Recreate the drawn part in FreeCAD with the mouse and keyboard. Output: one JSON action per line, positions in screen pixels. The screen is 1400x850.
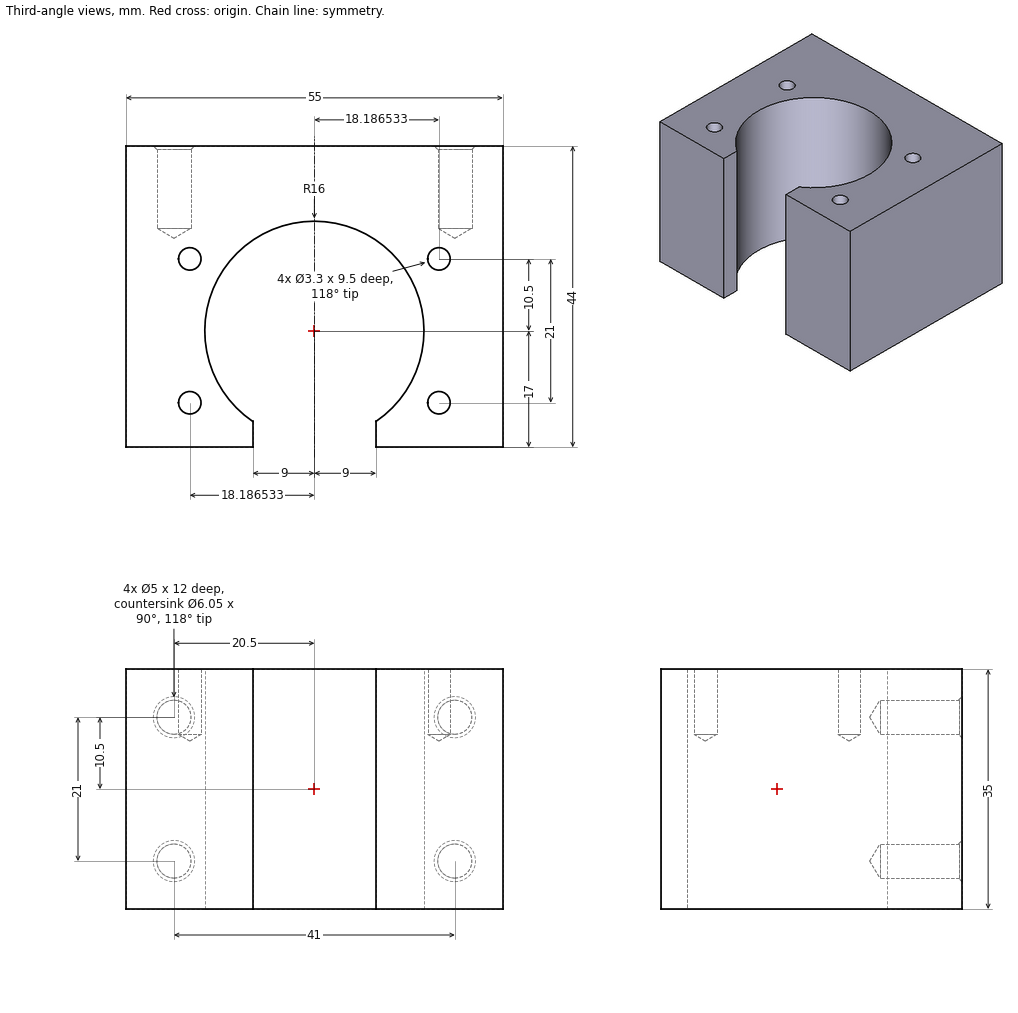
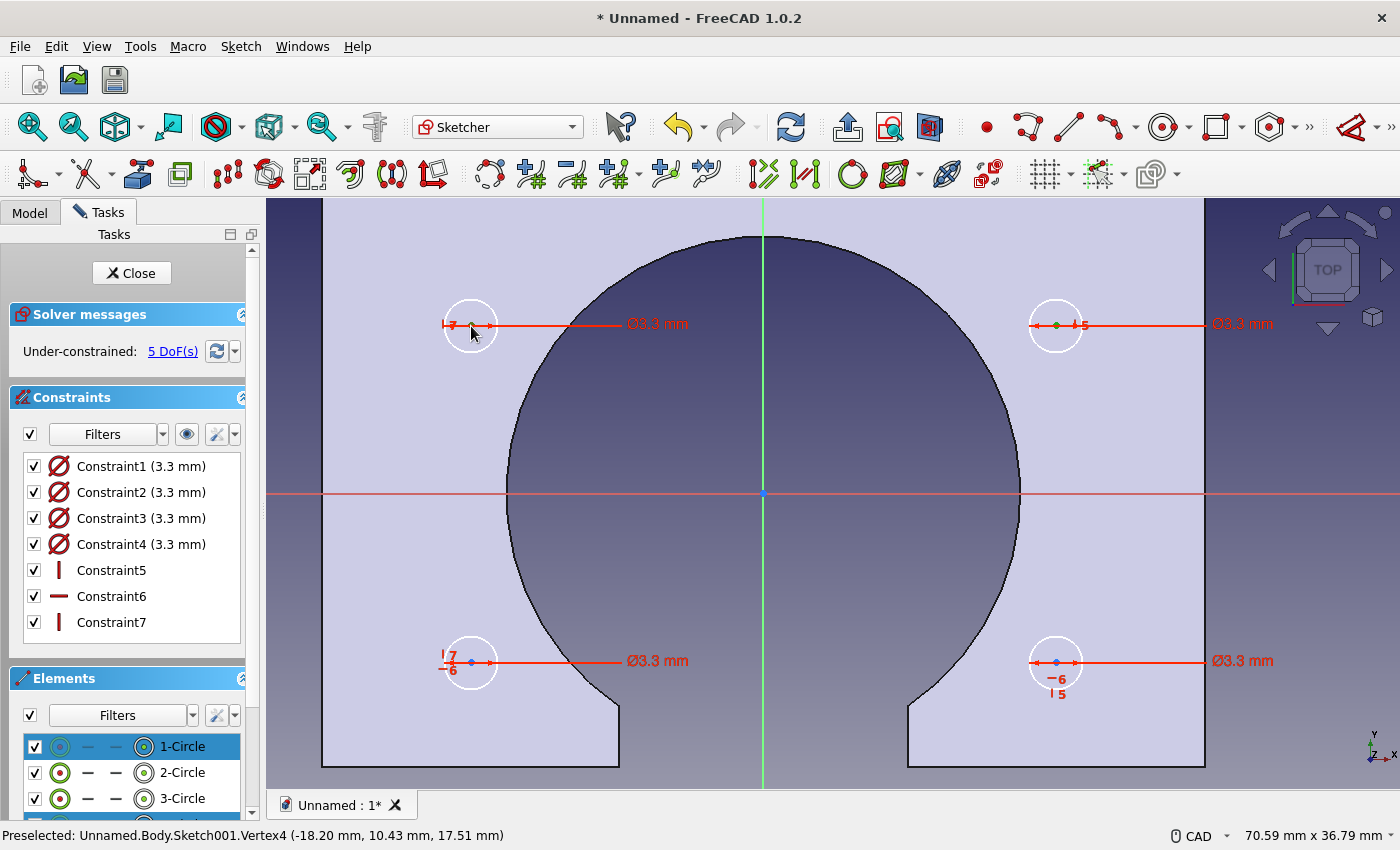
{"action": "key", "text": "h"}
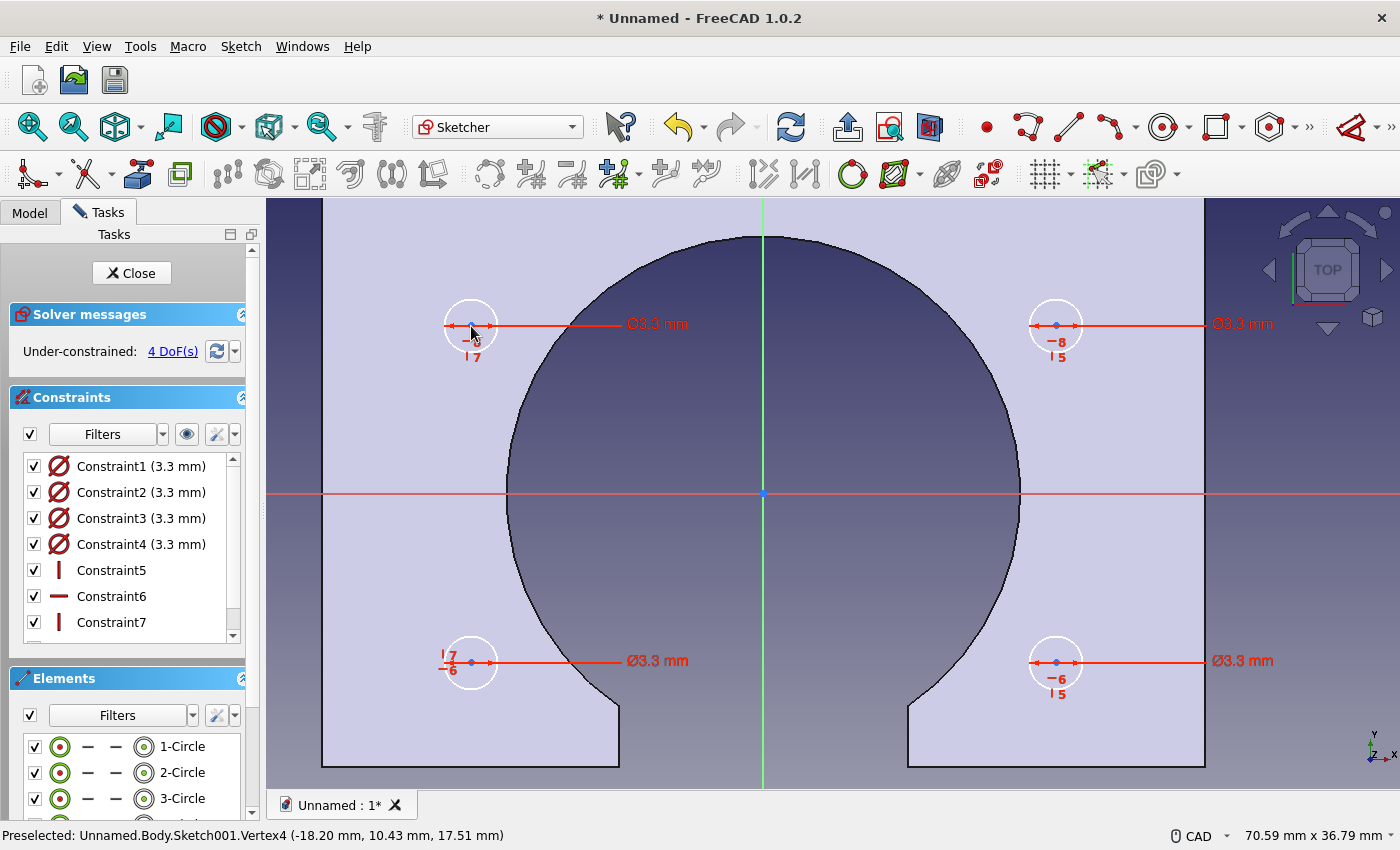
{"action": "left_click", "coordinate": [1350, 128]}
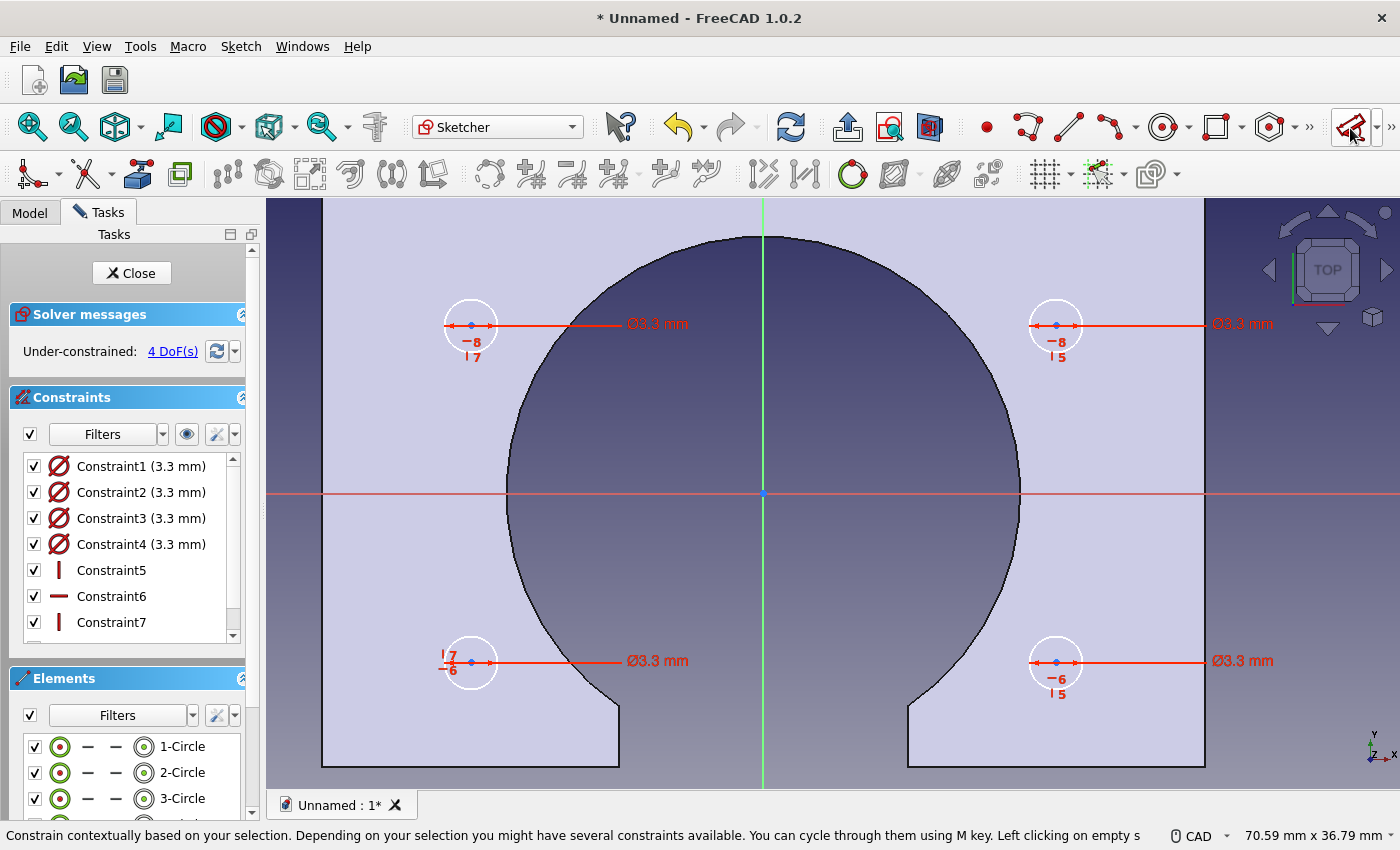
{"action": "left_click", "coordinate": [1056, 326]}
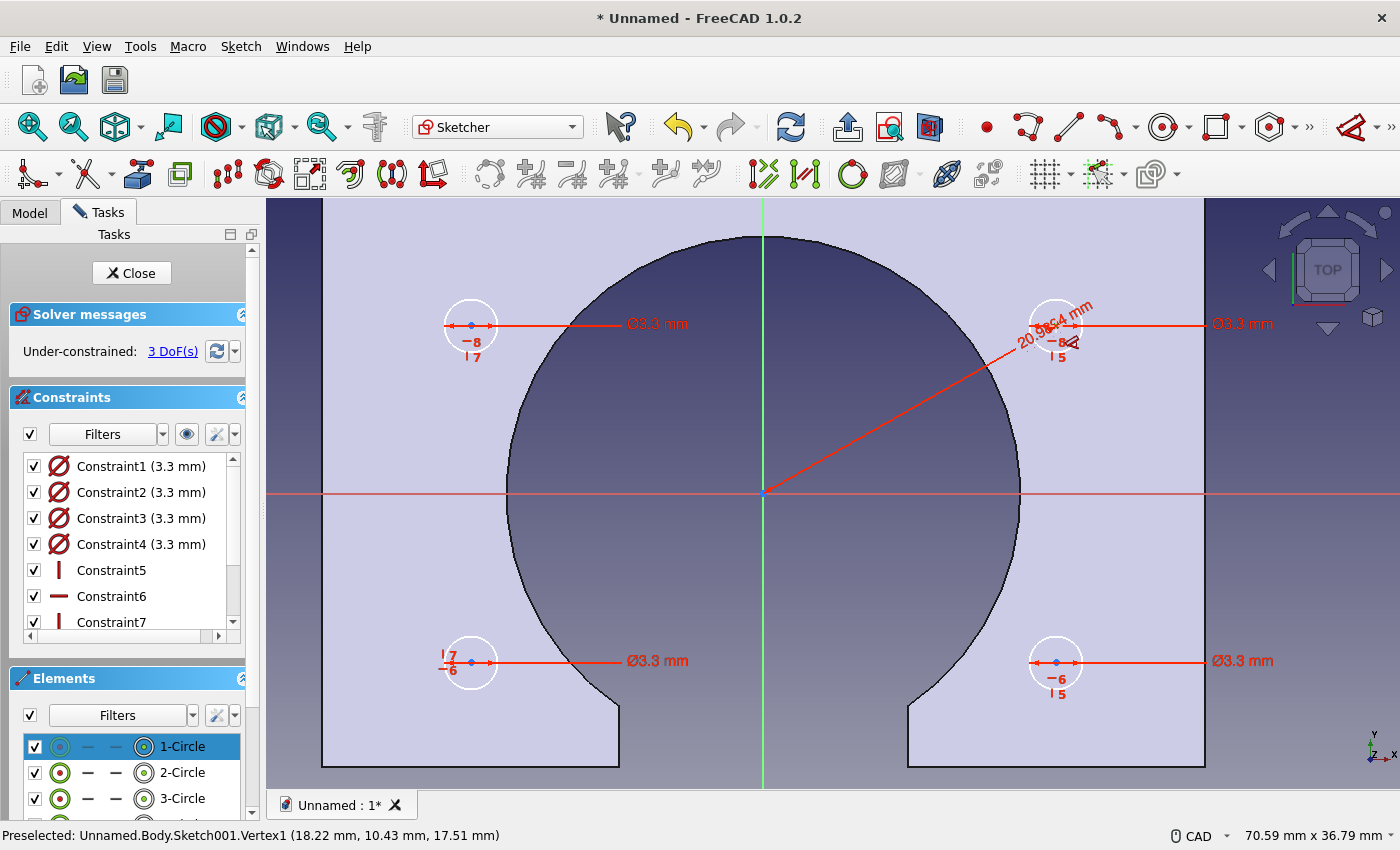
{"action": "left_click", "coordinate": [1056, 663]}
{"action": "left_click", "coordinate": [1090, 417]}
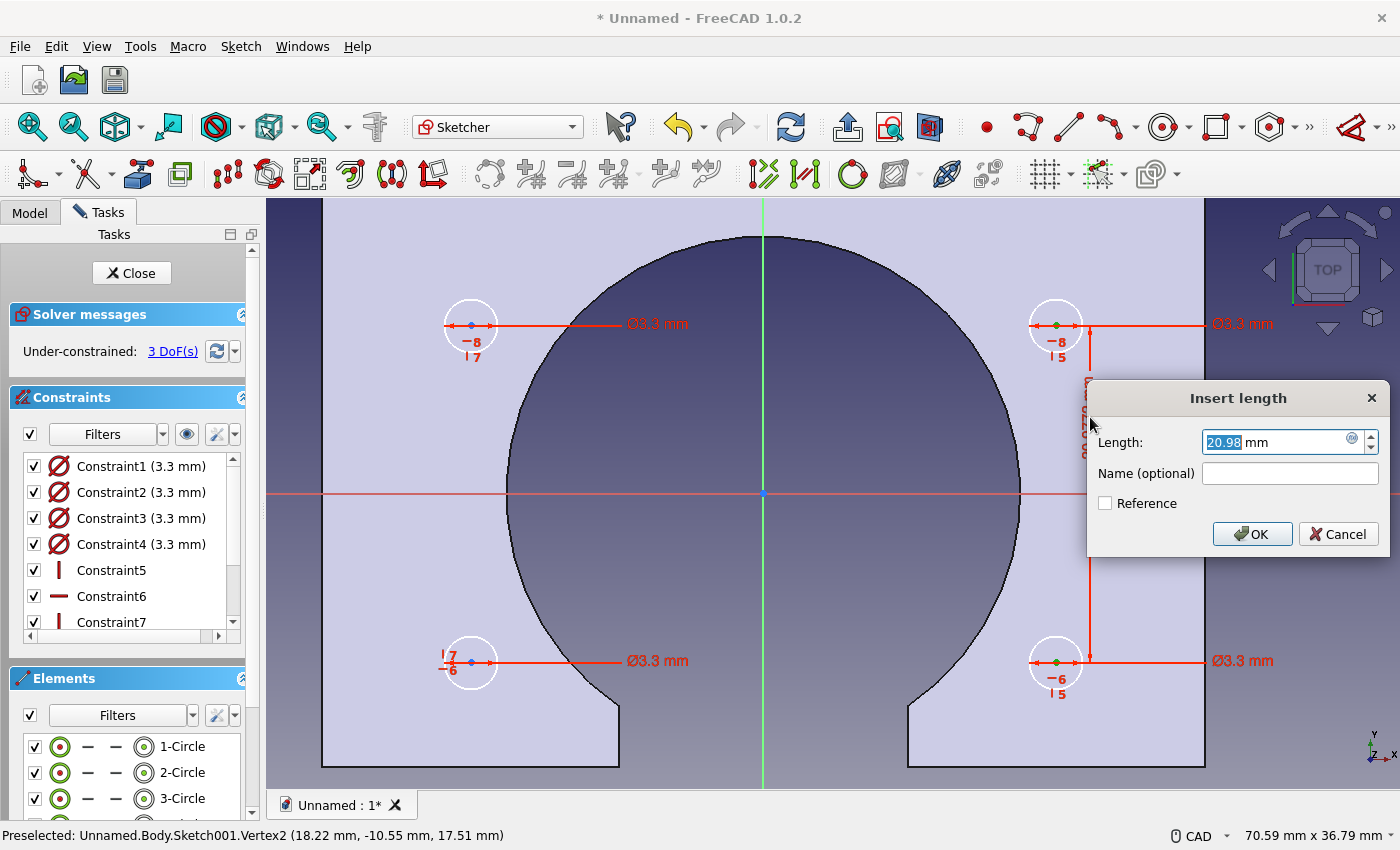
{"action": "type", "text": "21"}
{"action": "key", "text": "Return"}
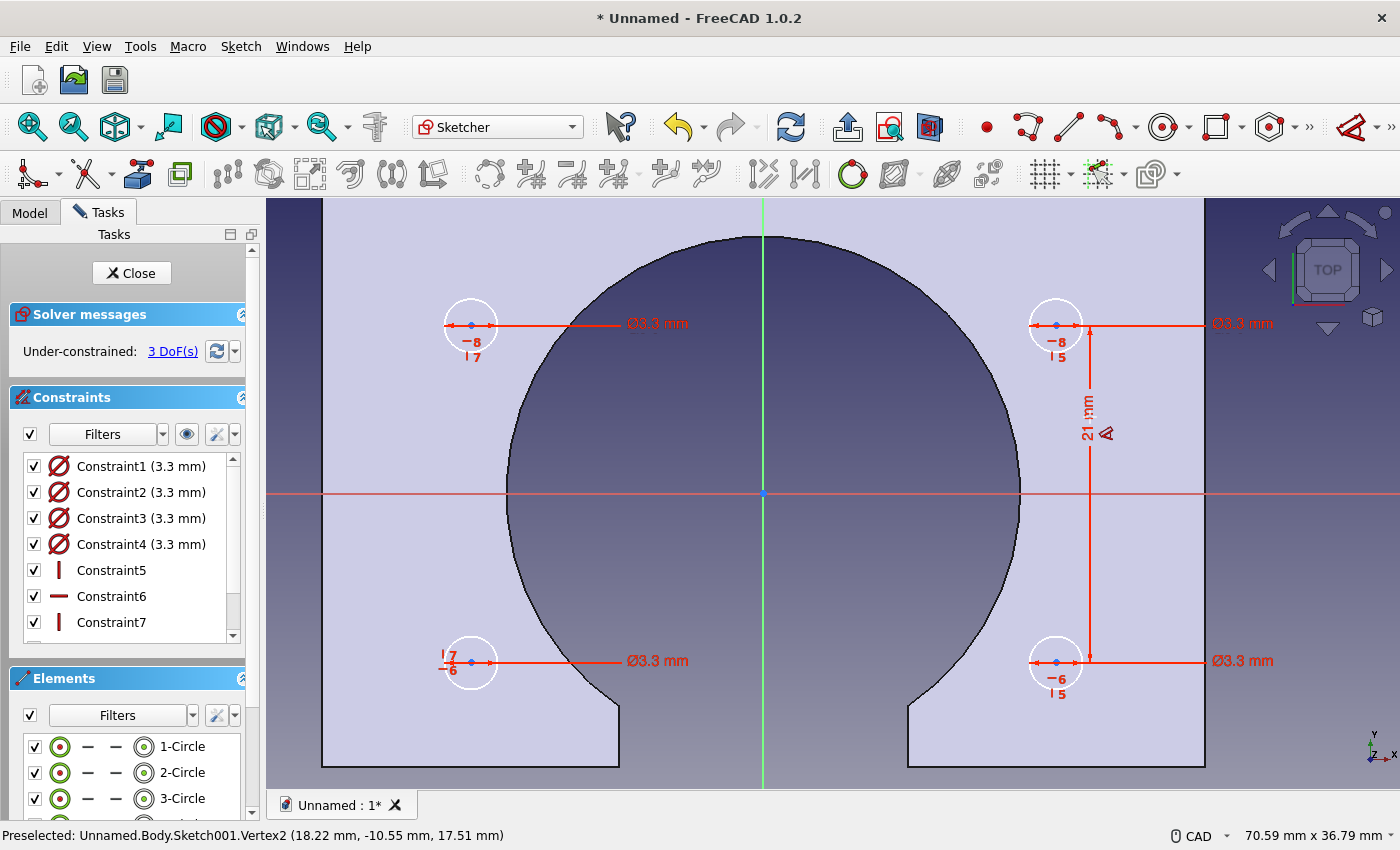
{"action": "left_click", "coordinate": [1056, 326]}
{"action": "left_click", "coordinate": [1090, 371]}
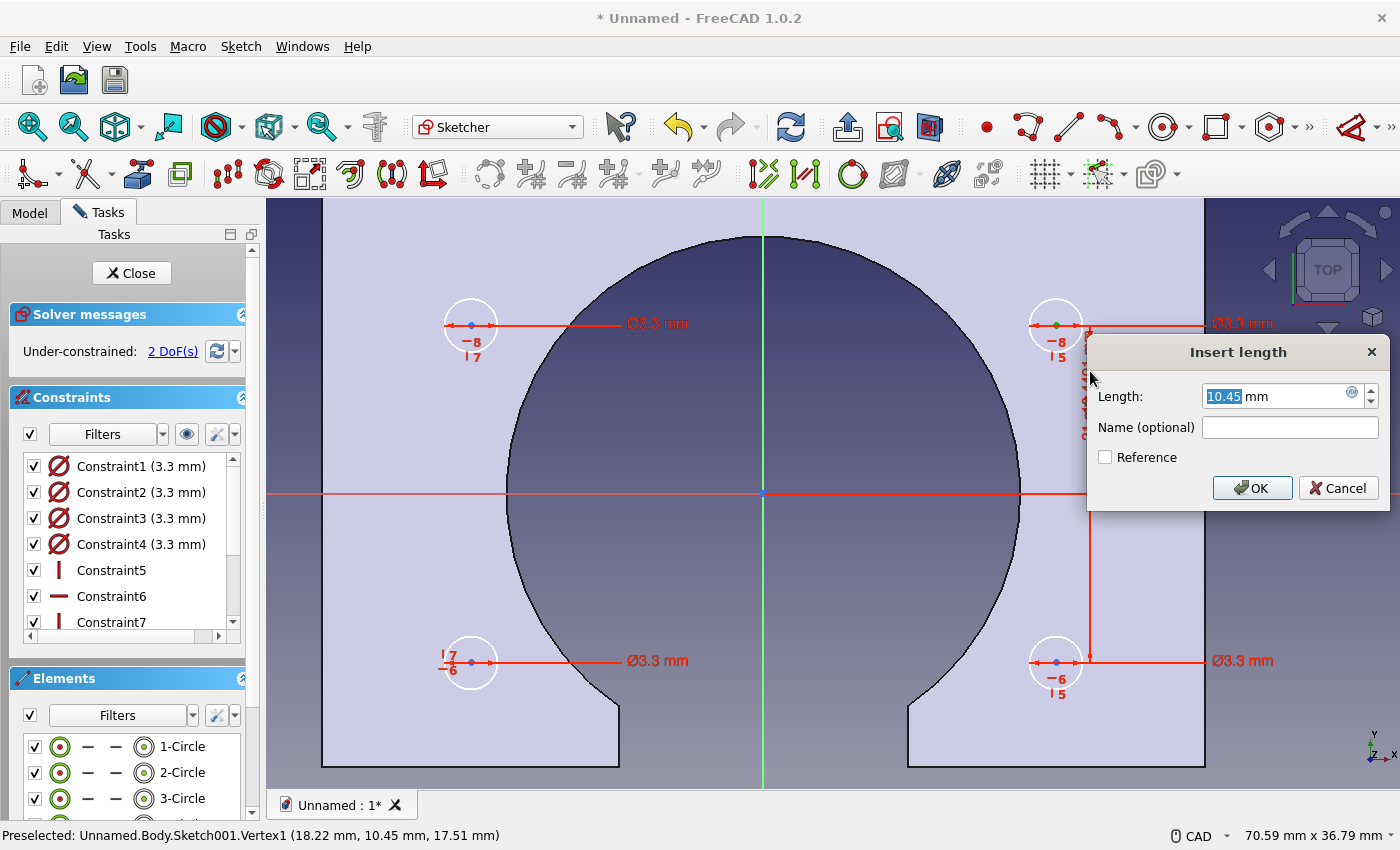
{"action": "type", "text": "10.5"}
{"action": "key", "text": "Return"}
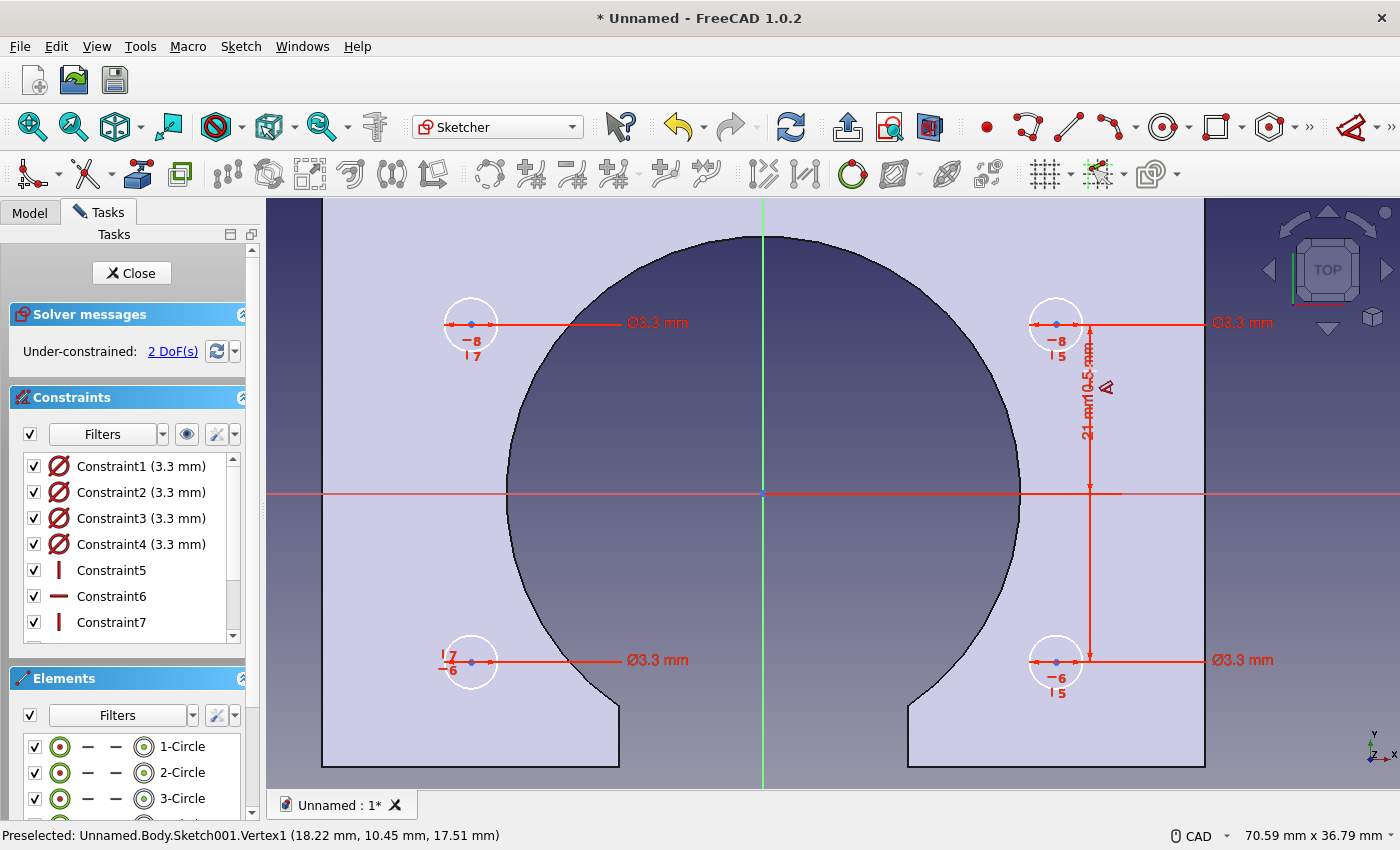
{"action": "left_click", "coordinate": [1056, 325]}
{"action": "left_click", "coordinate": [910, 291]}